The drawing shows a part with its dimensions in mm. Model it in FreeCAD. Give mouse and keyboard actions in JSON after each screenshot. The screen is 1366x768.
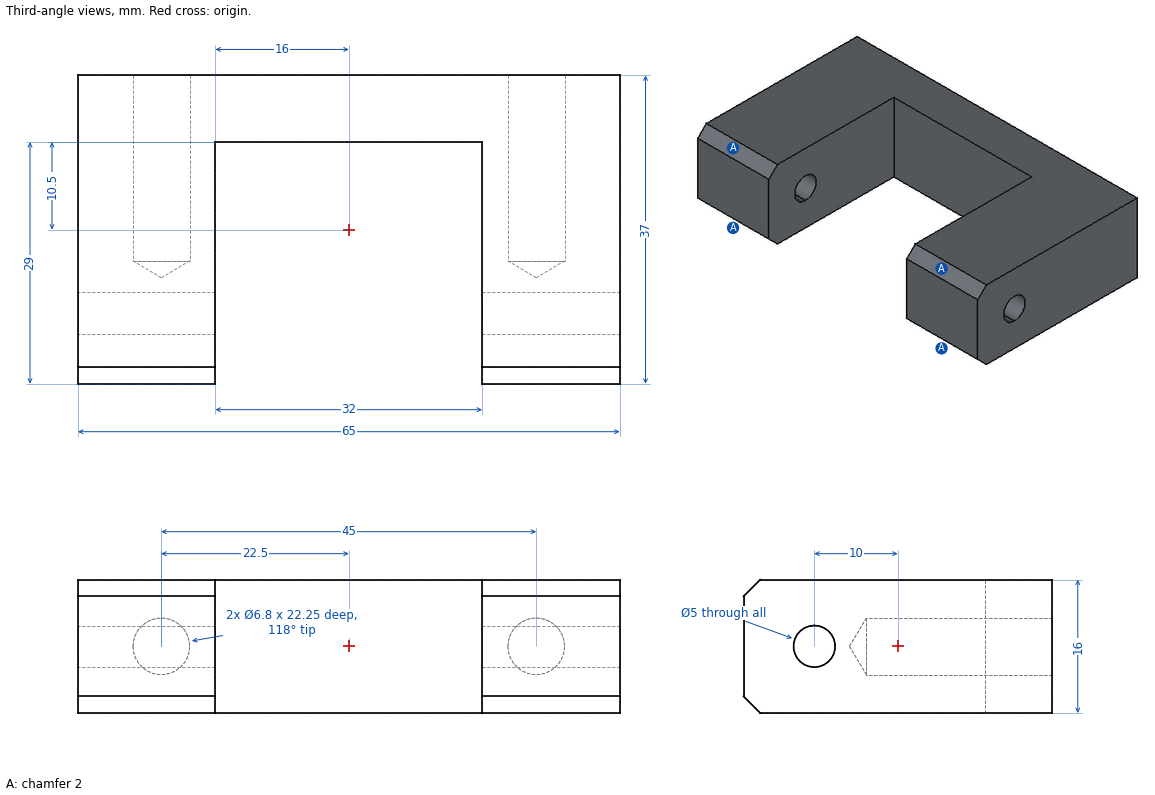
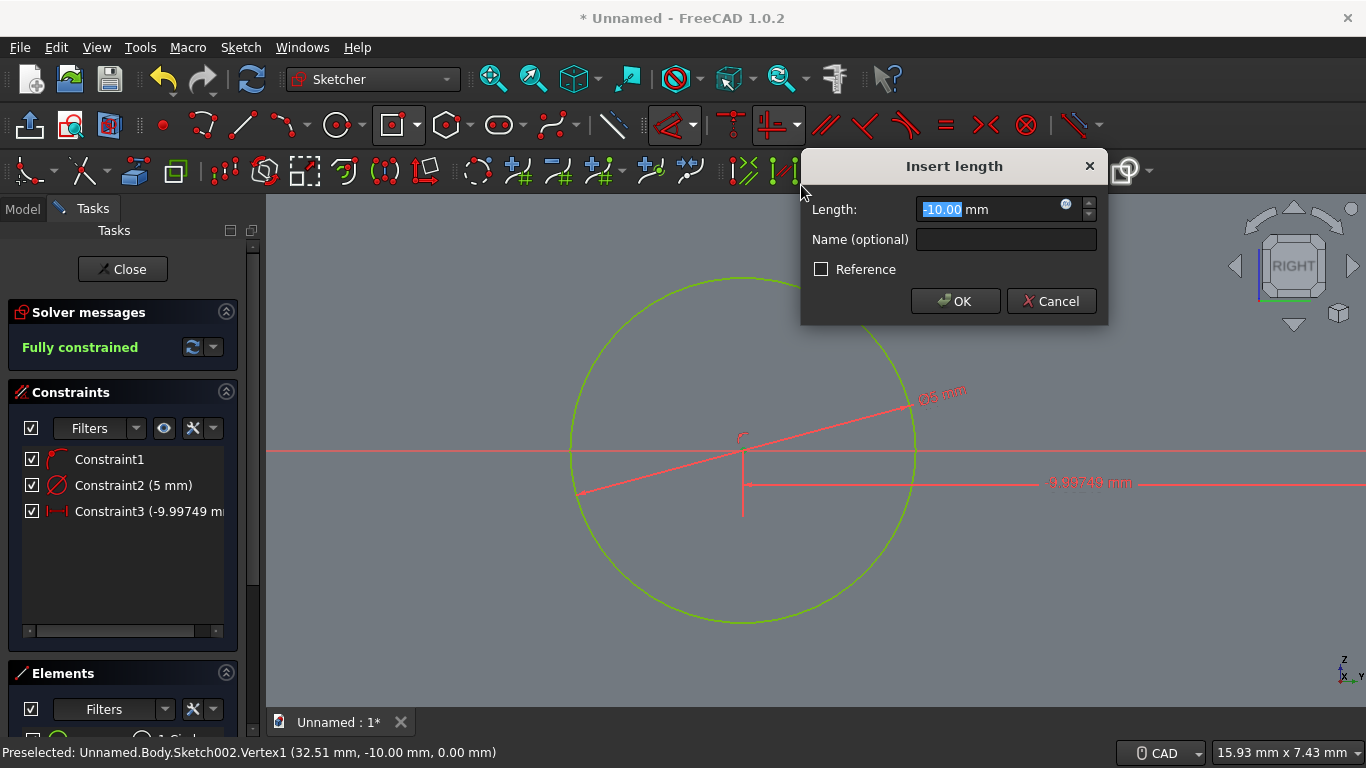
{"action": "type", "text": "-10"}
{"action": "key", "text": "Return"}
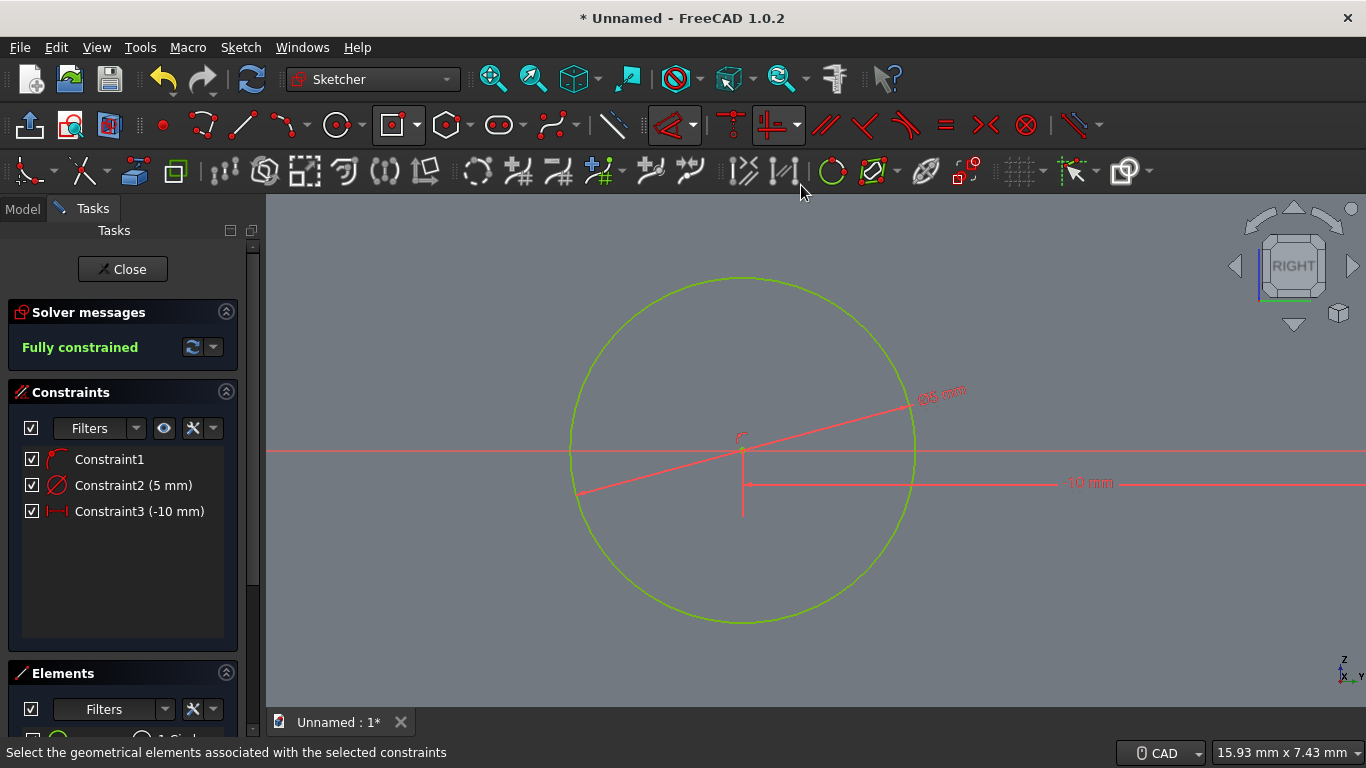
{"action": "left_click", "coordinate": [123, 269]}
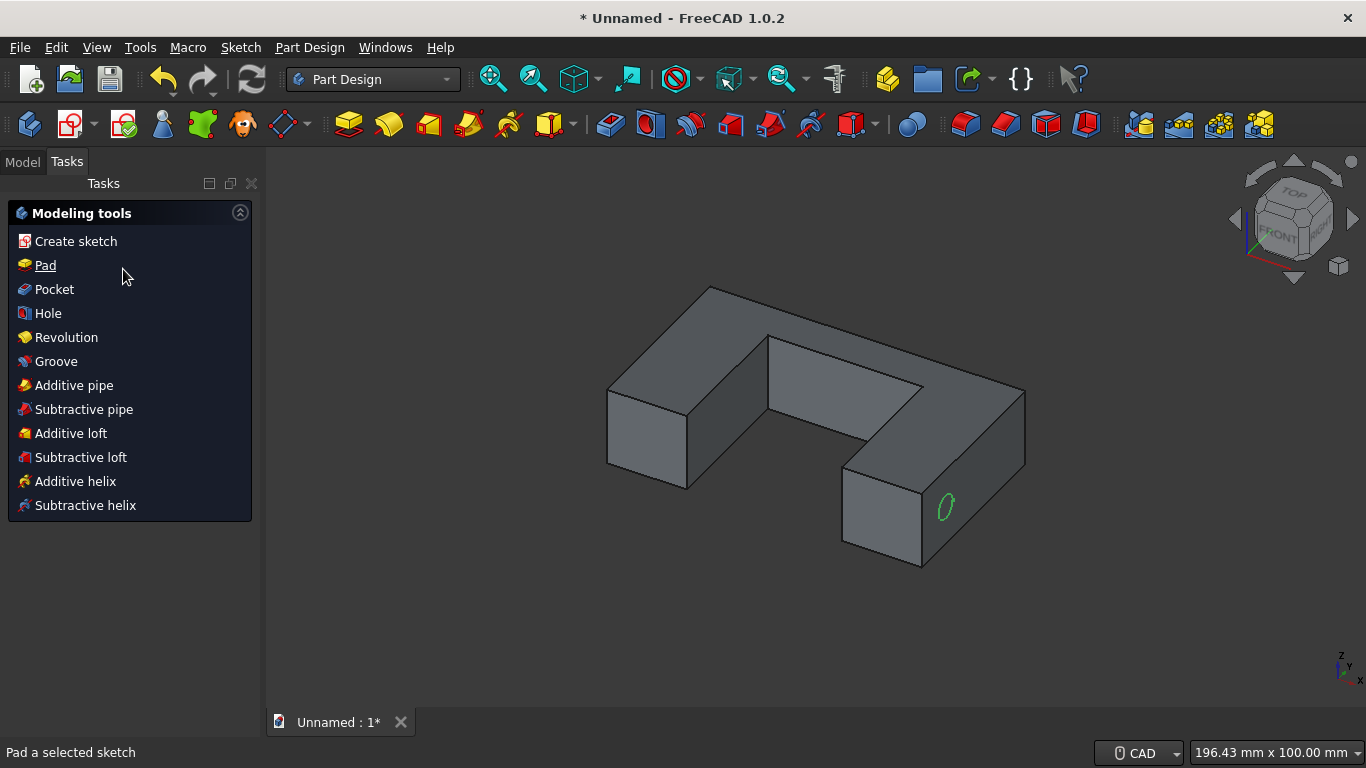
{"action": "left_click", "coordinate": [652, 124]}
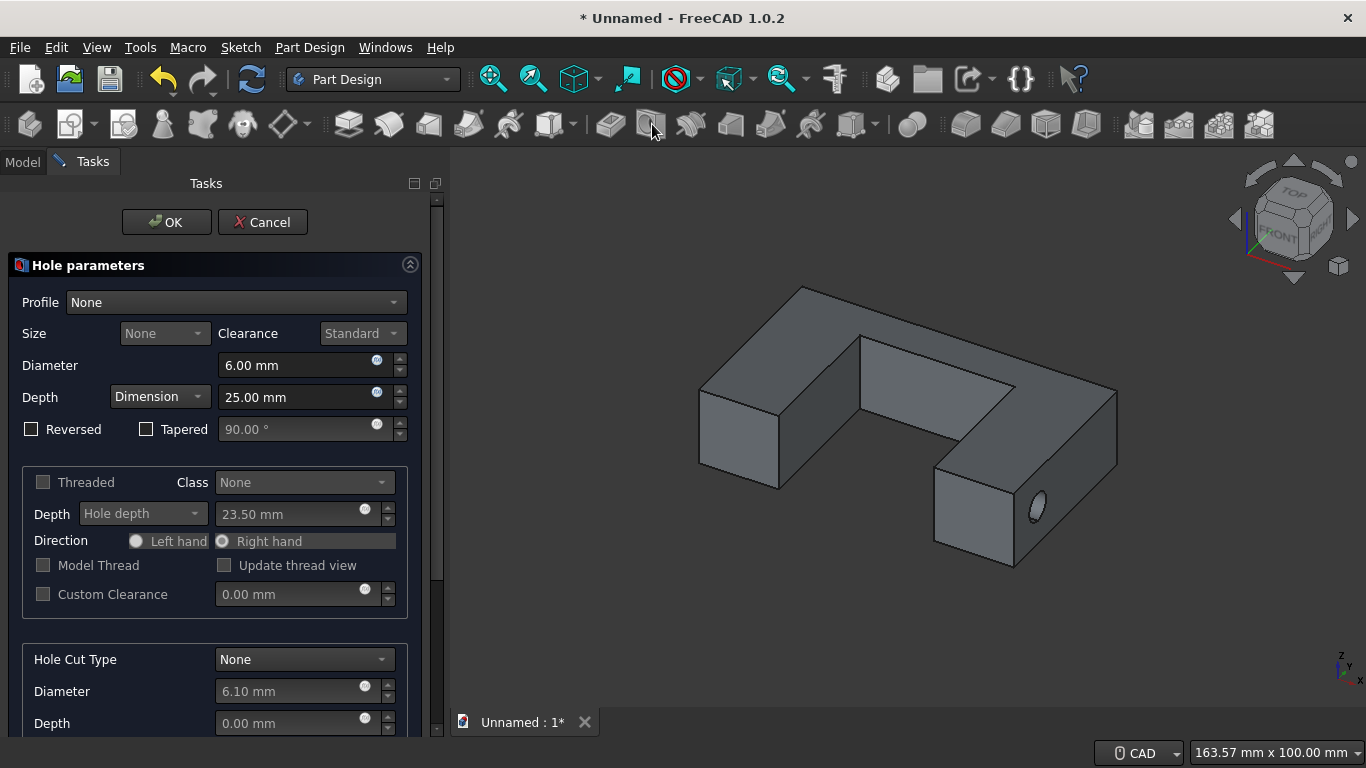
{"action": "triple_click", "coordinate": [305, 365]}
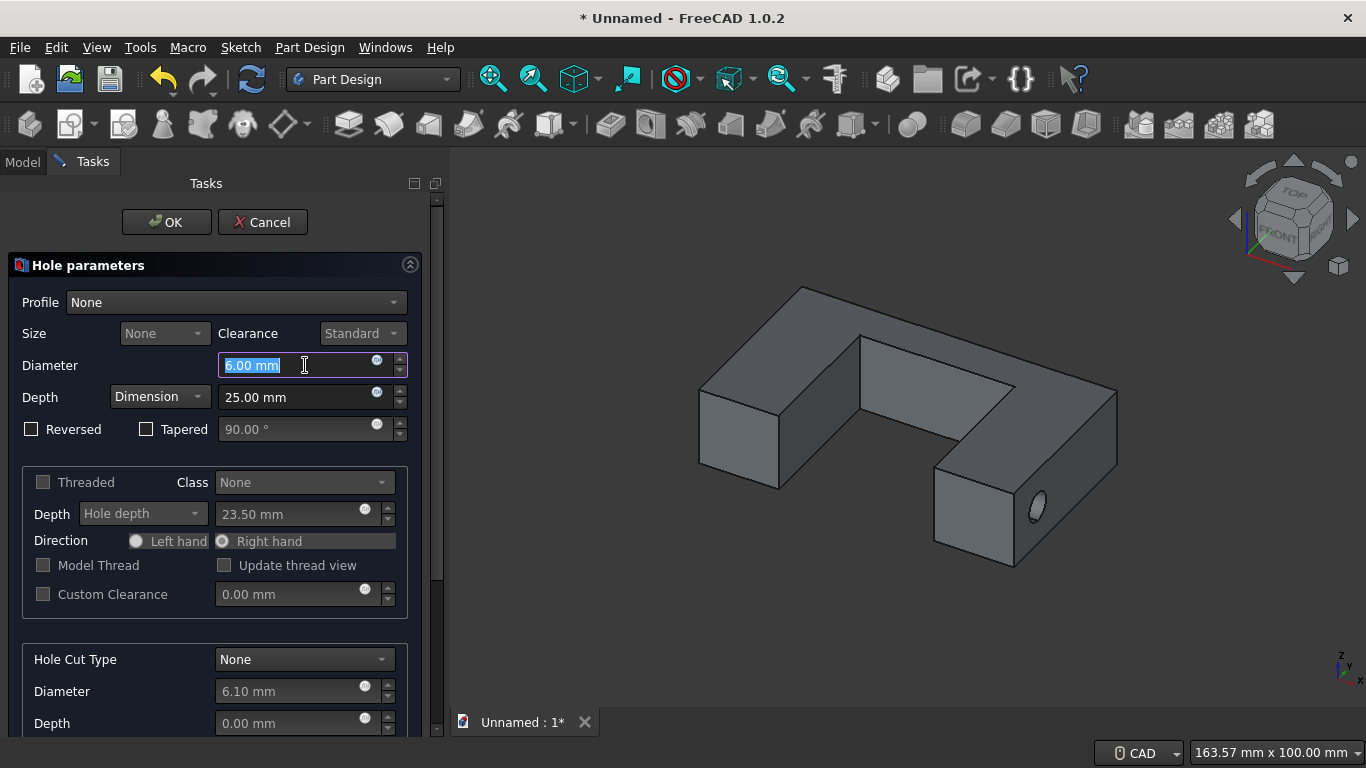
{"action": "type", "text": "5"}
{"action": "key", "text": "Tab"}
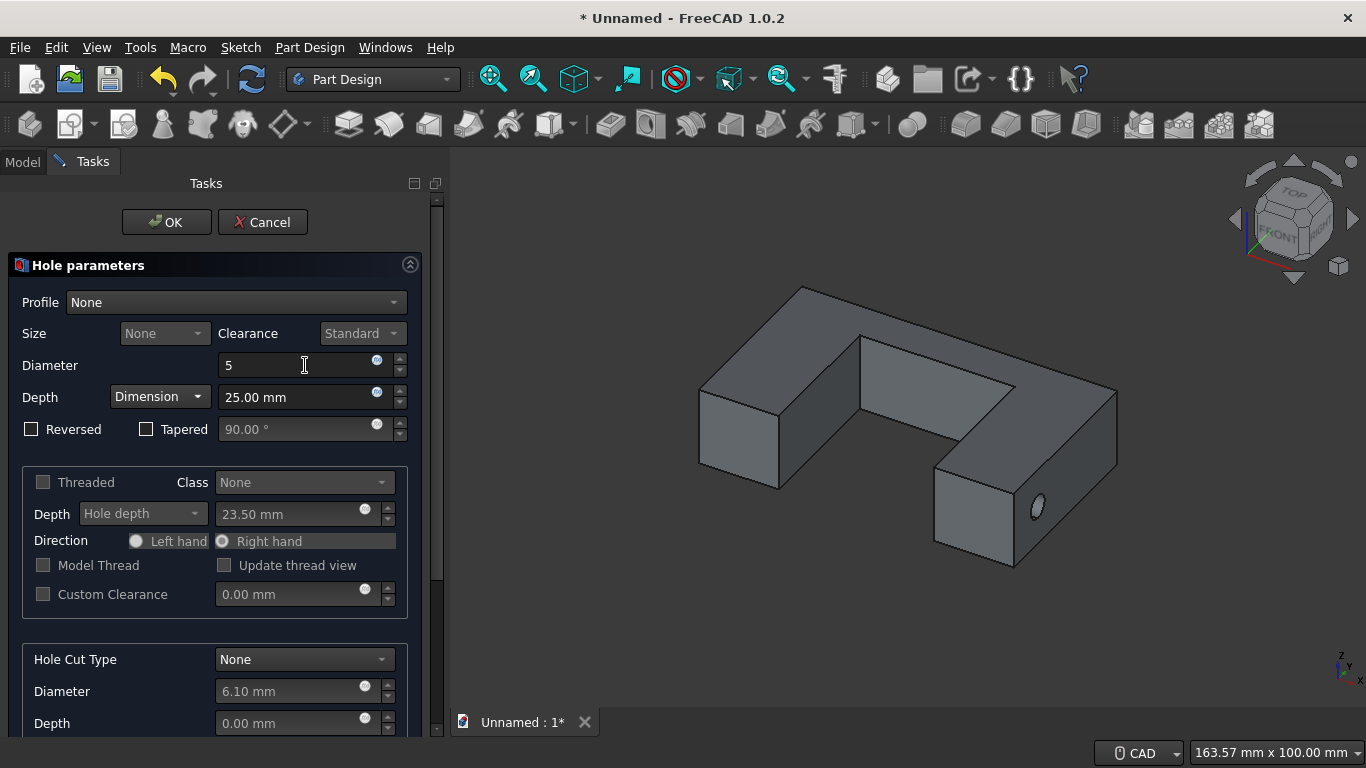
{"action": "left_click", "coordinate": [161, 396]}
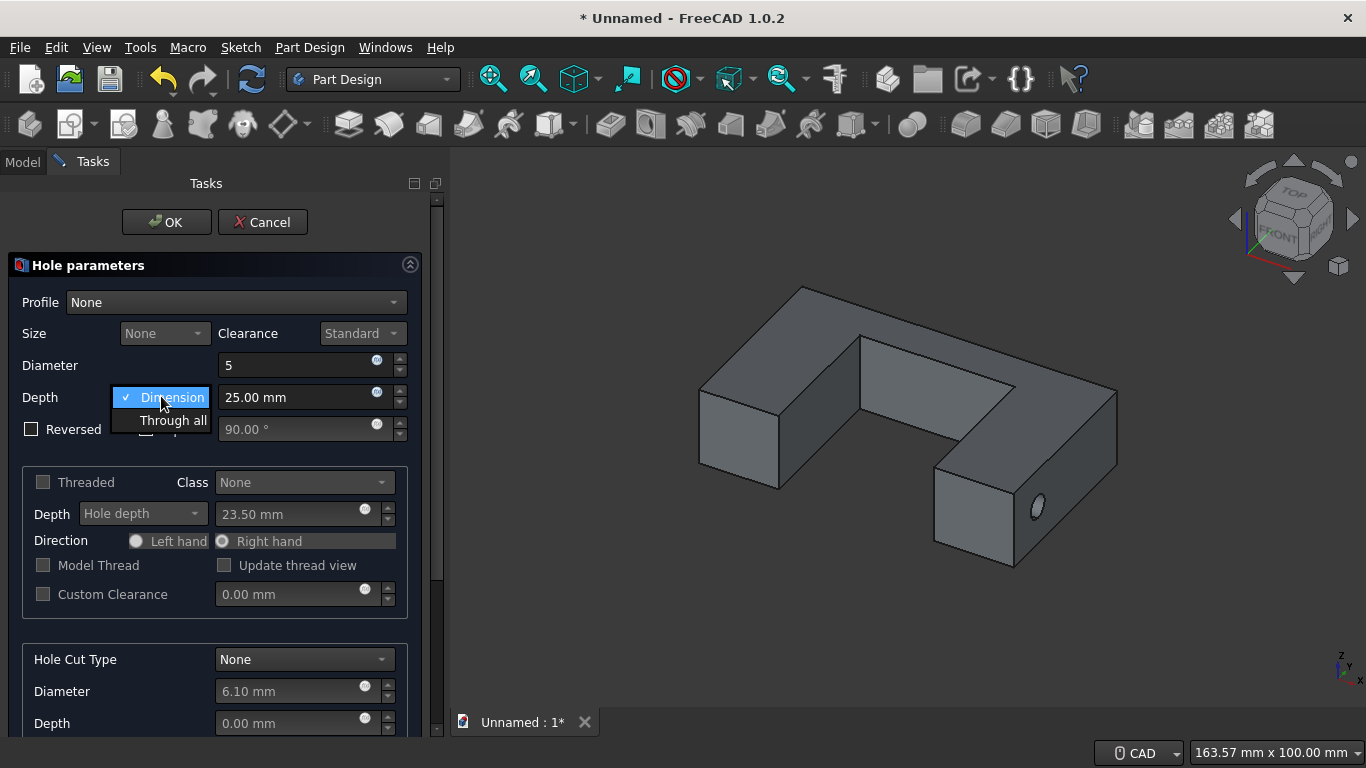
{"action": "left_click", "coordinate": [160, 420]}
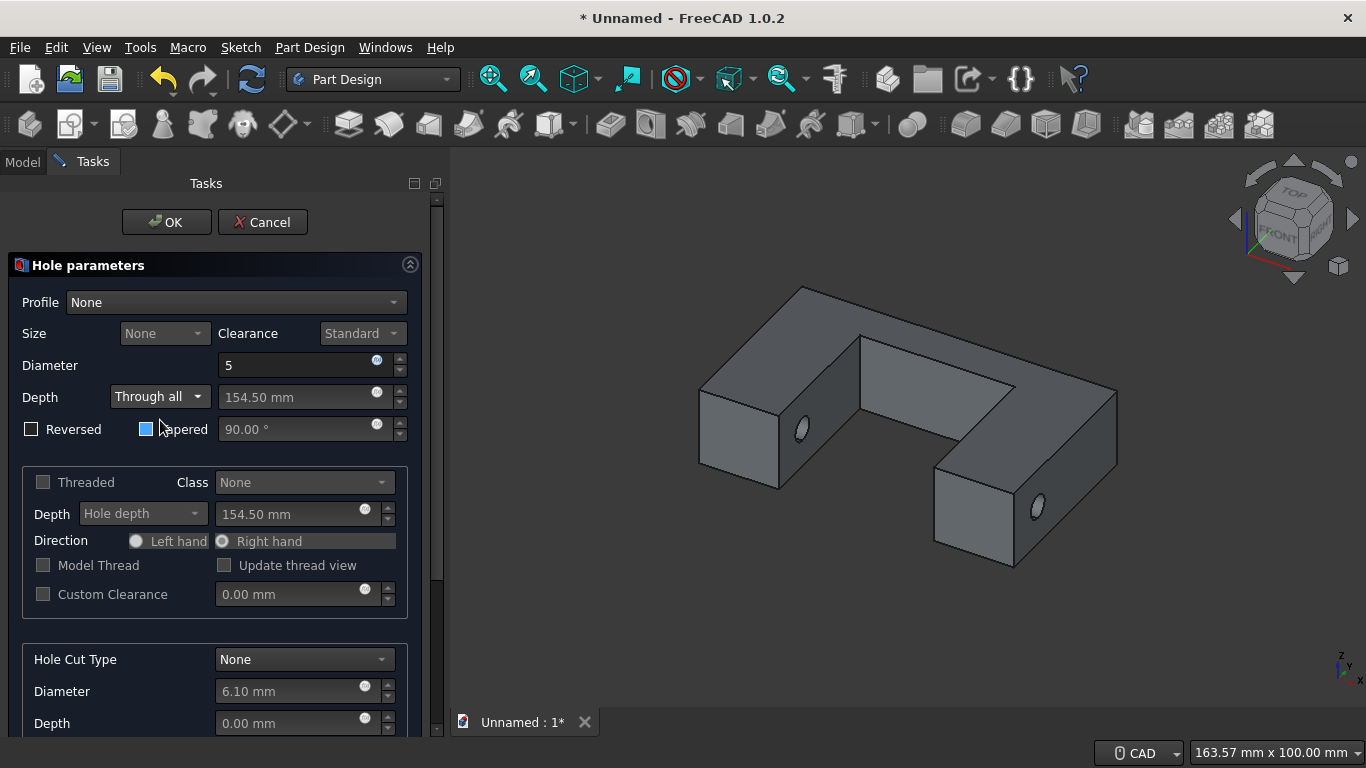
{"action": "left_click", "coordinate": [167, 222]}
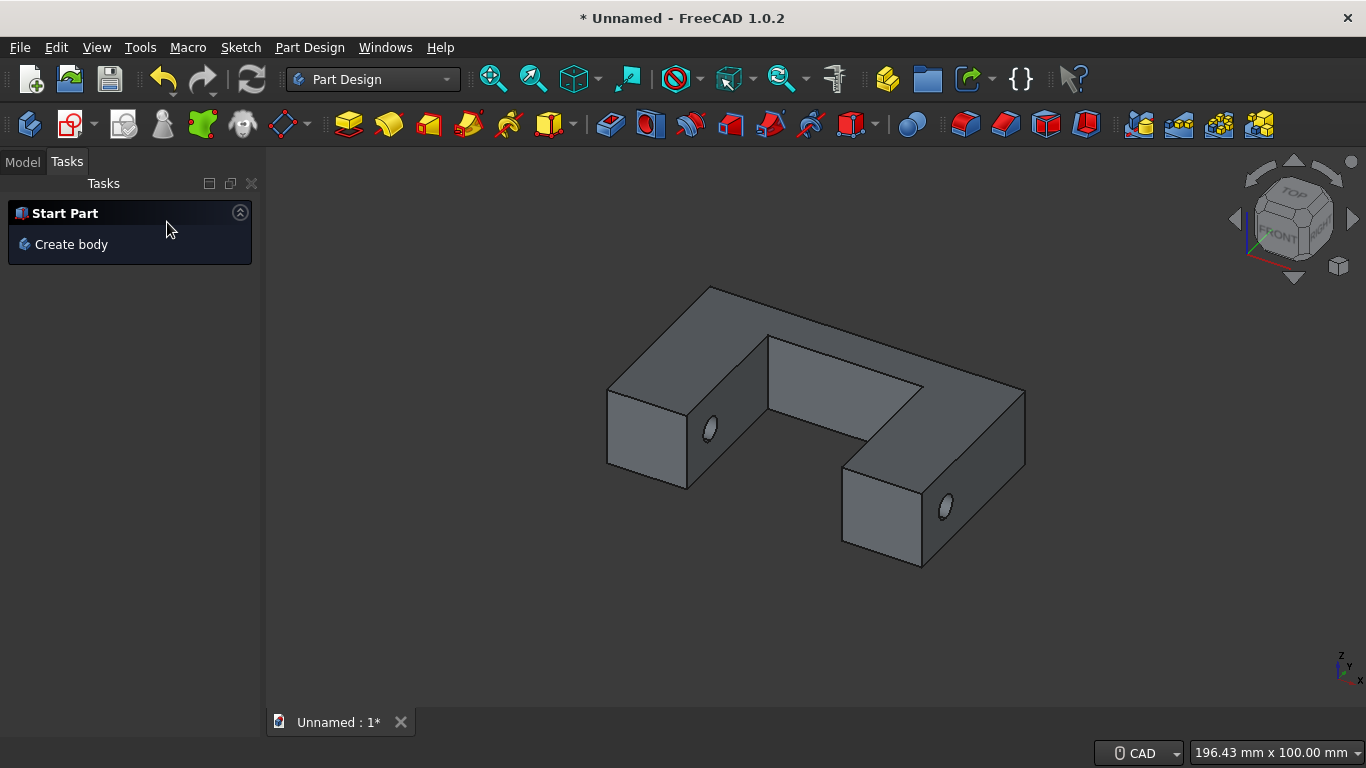
{"action": "key", "text": "4"}